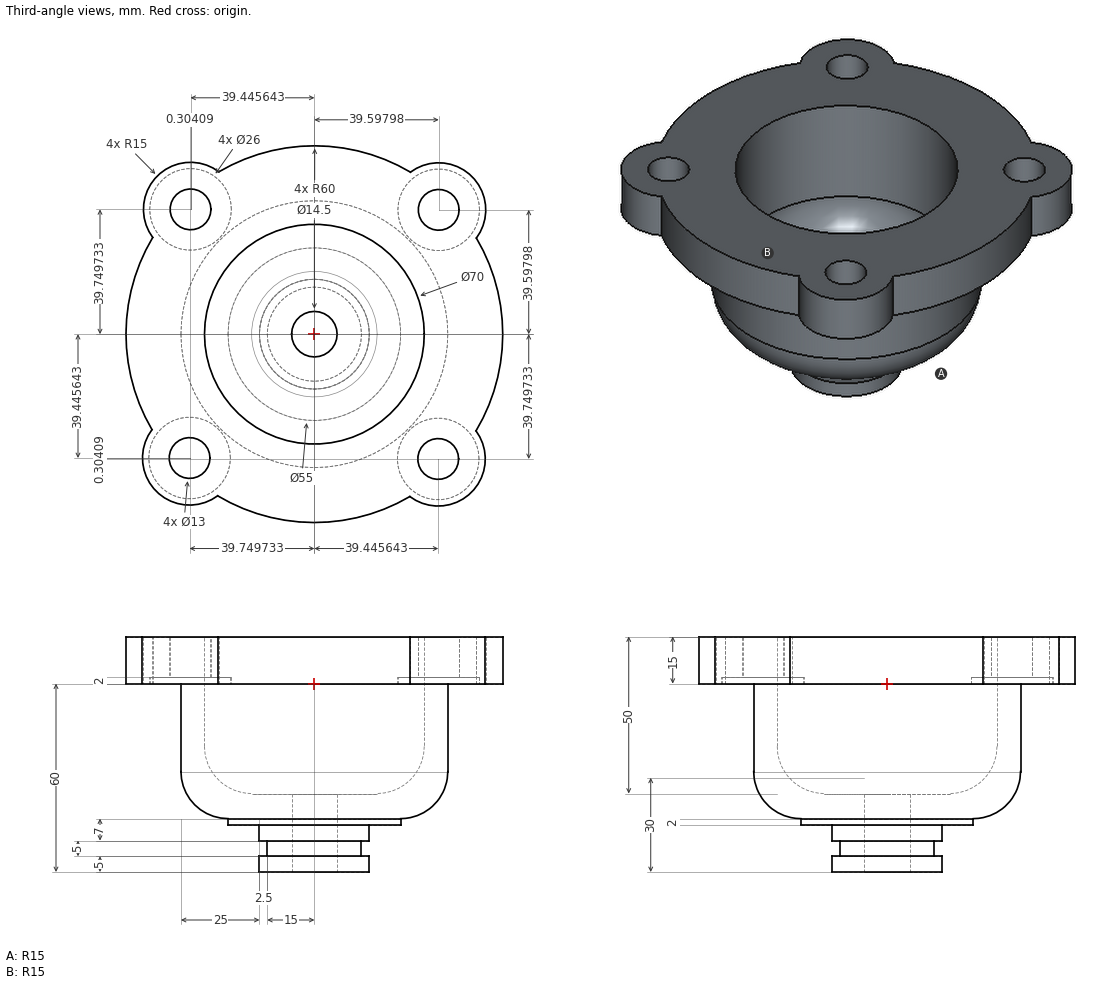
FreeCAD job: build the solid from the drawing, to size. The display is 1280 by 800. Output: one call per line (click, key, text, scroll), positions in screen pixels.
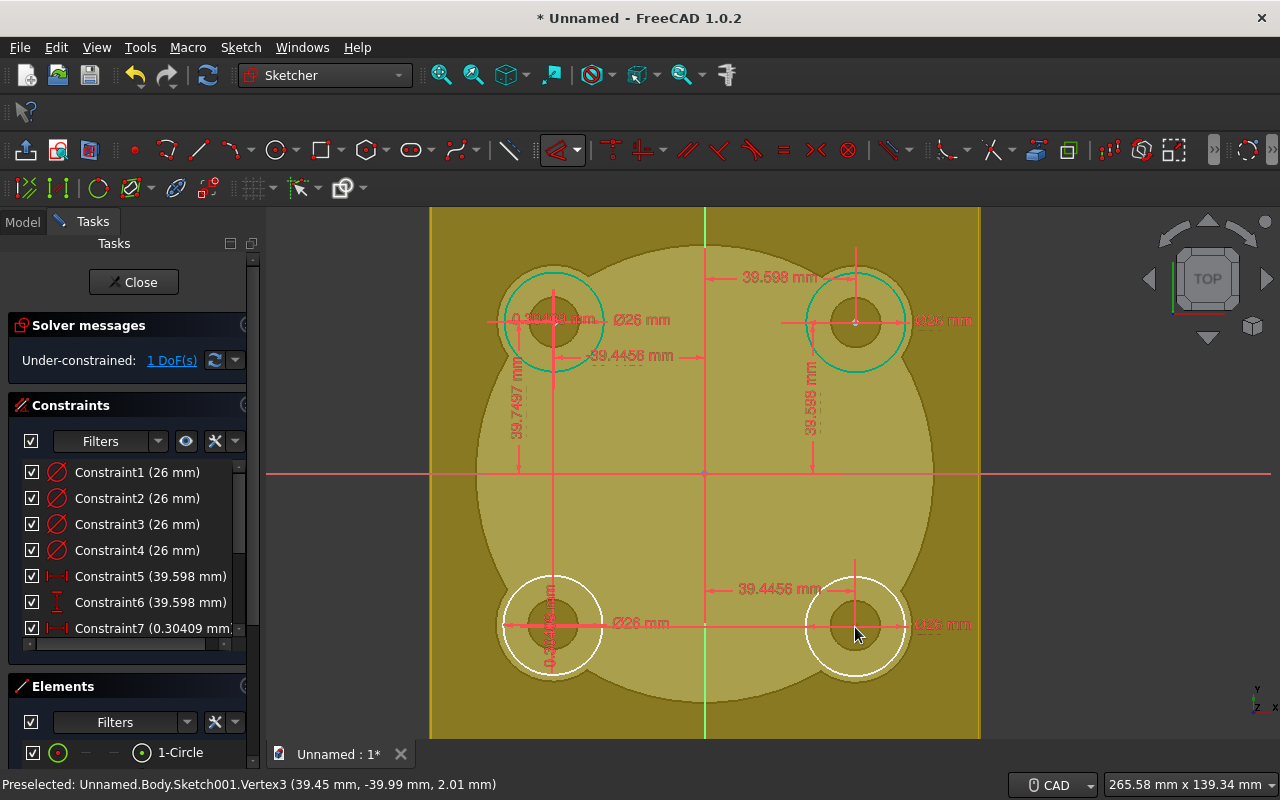
click(580, 150)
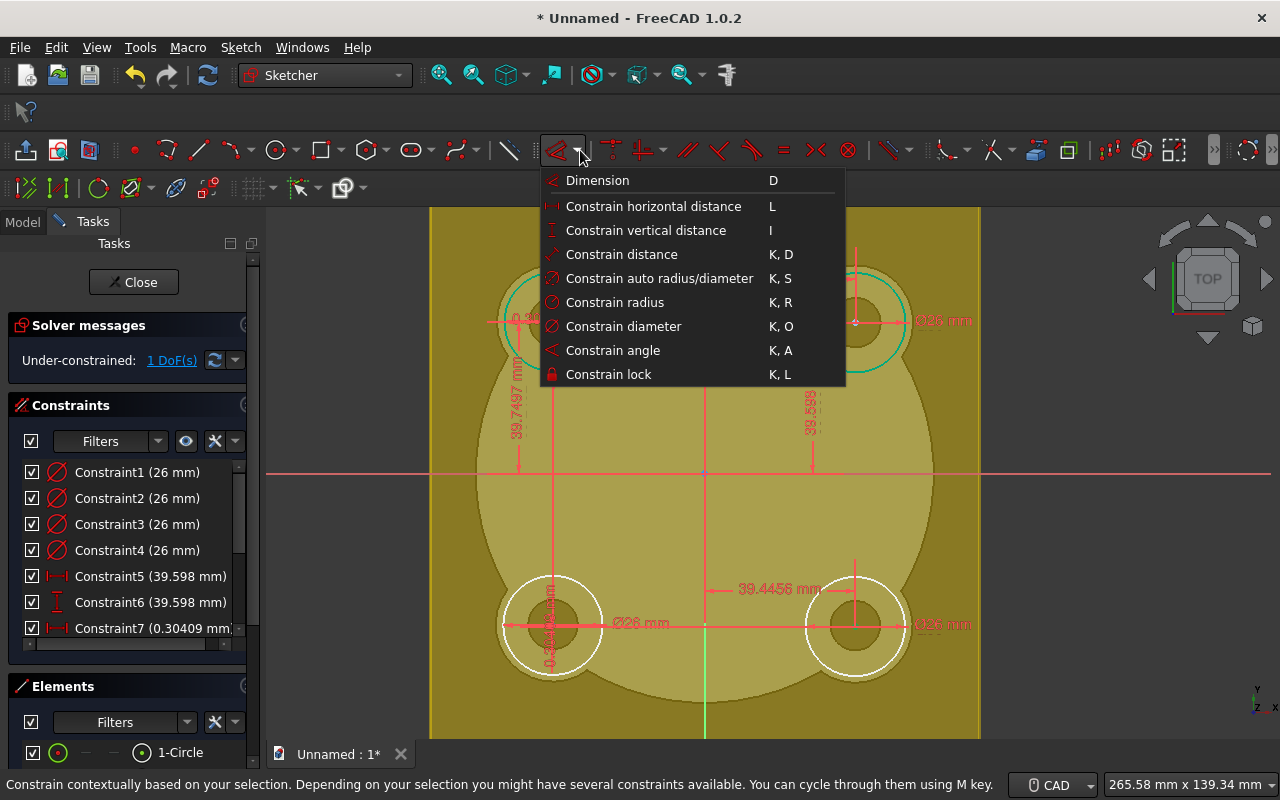
click(693, 230)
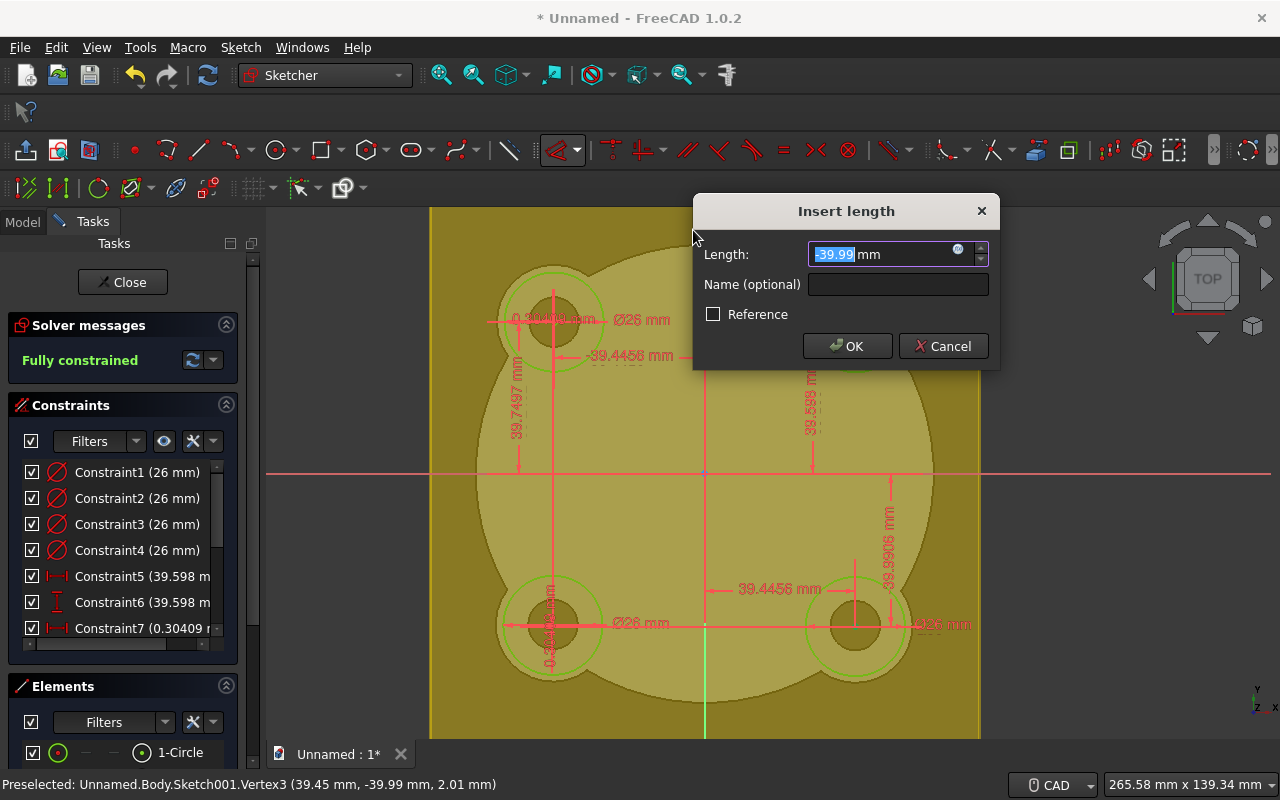
text(-39.749733)
key(Return)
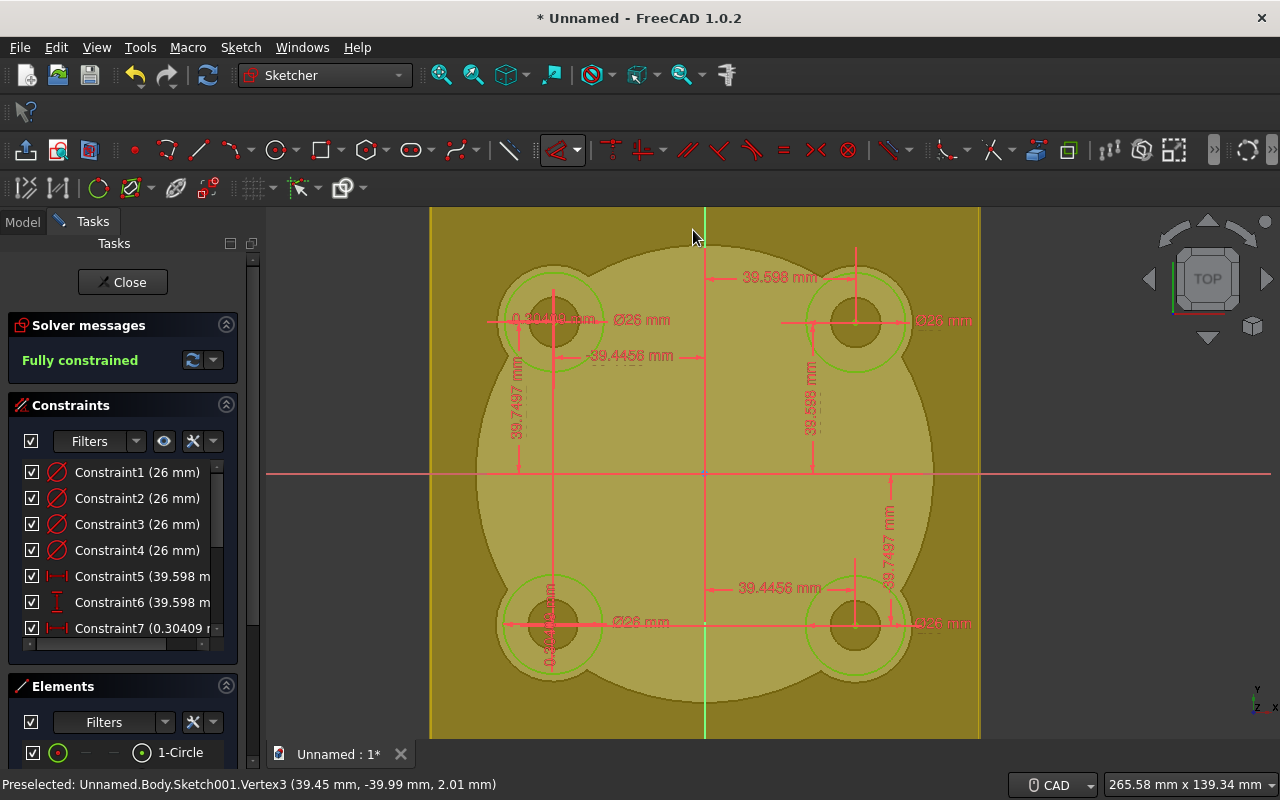
click(123, 282)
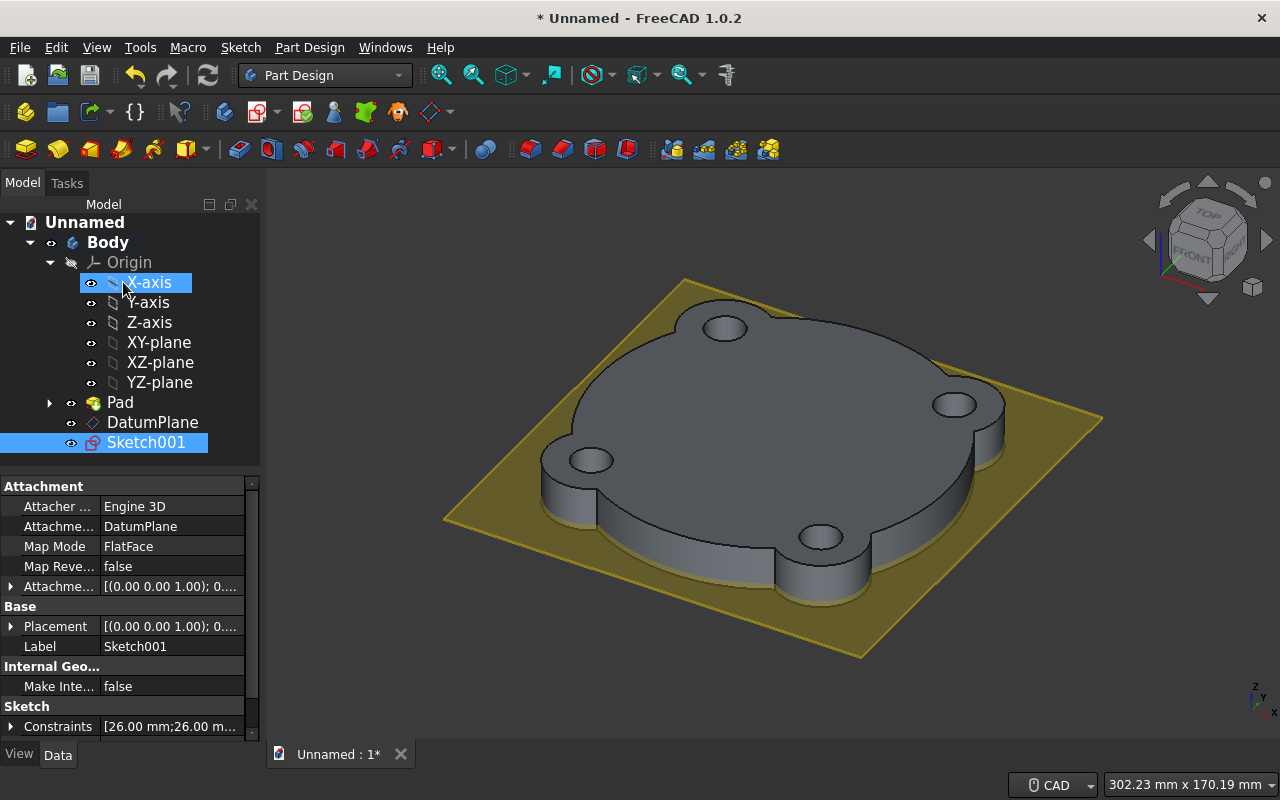
click(240, 150)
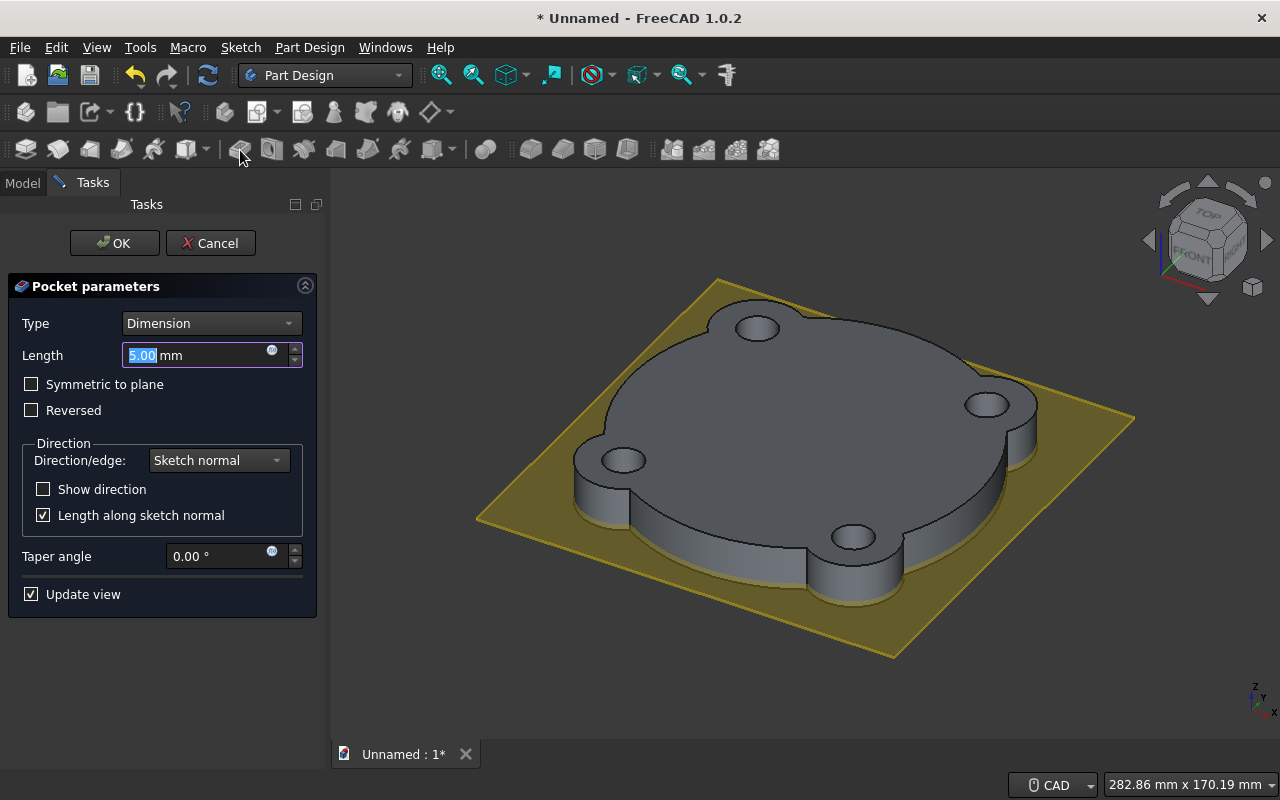
text(2)
key(Tab)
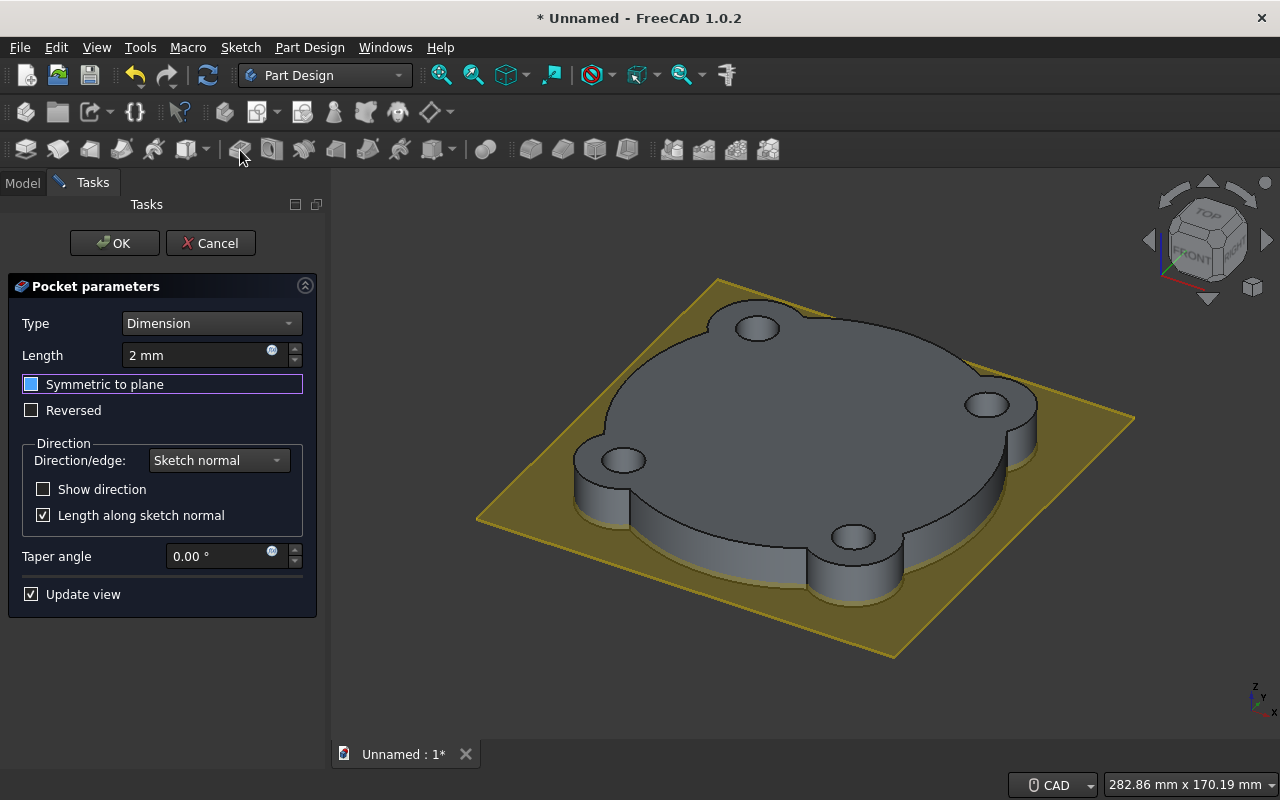
click(115, 243)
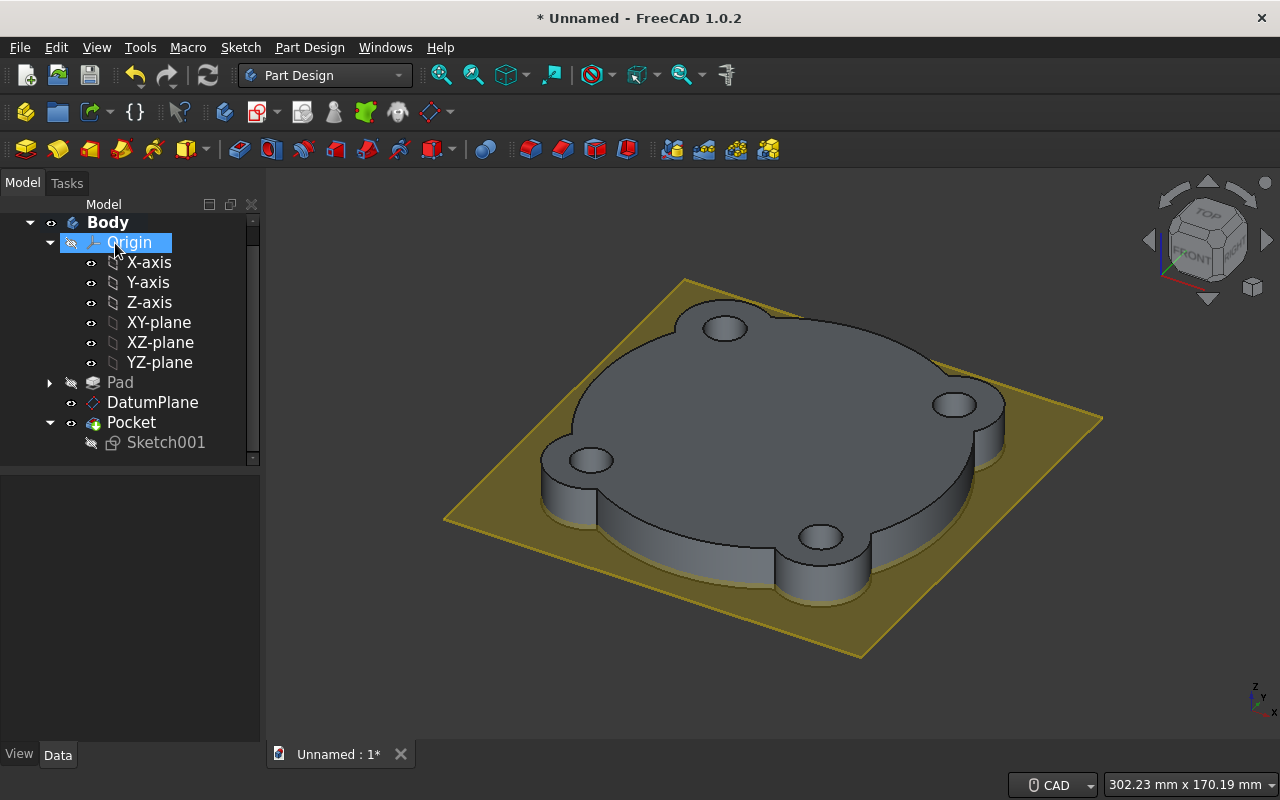
click(116, 403)
key(space)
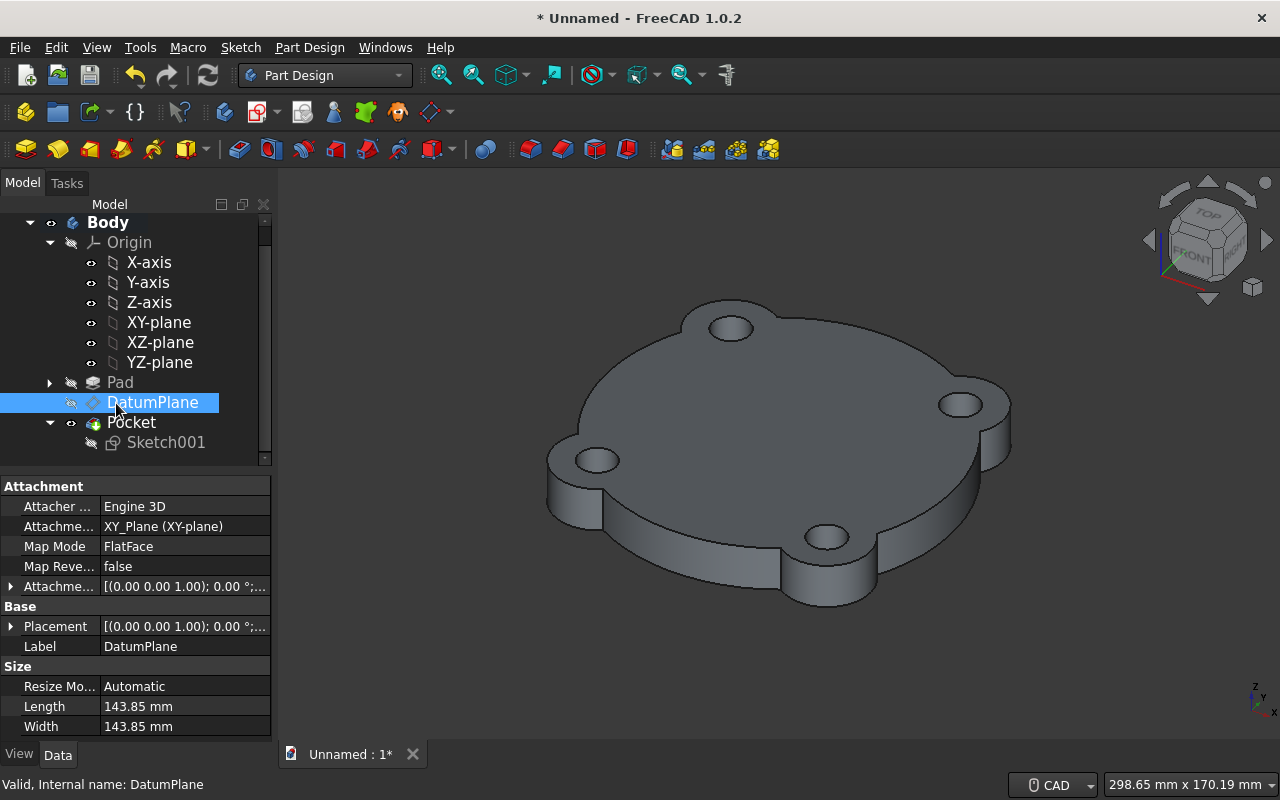
click(318, 699)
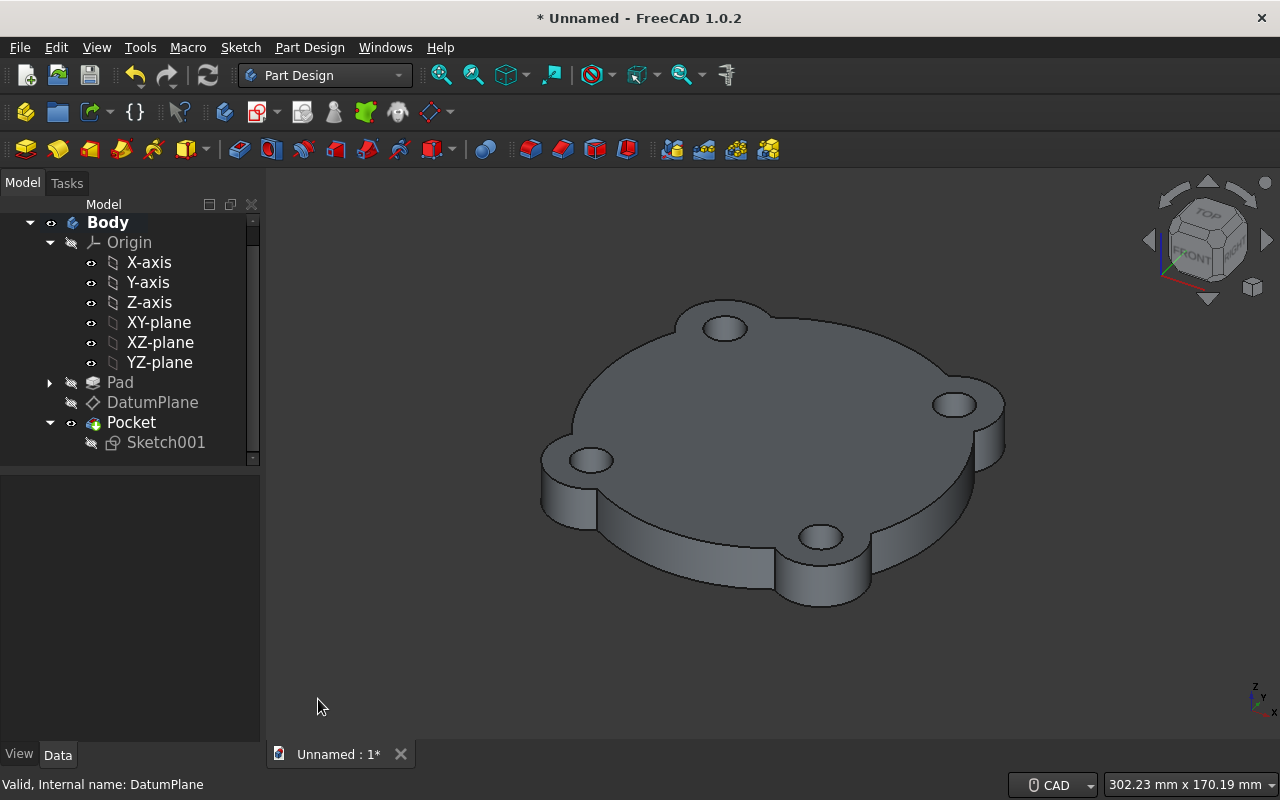
click(258, 112)